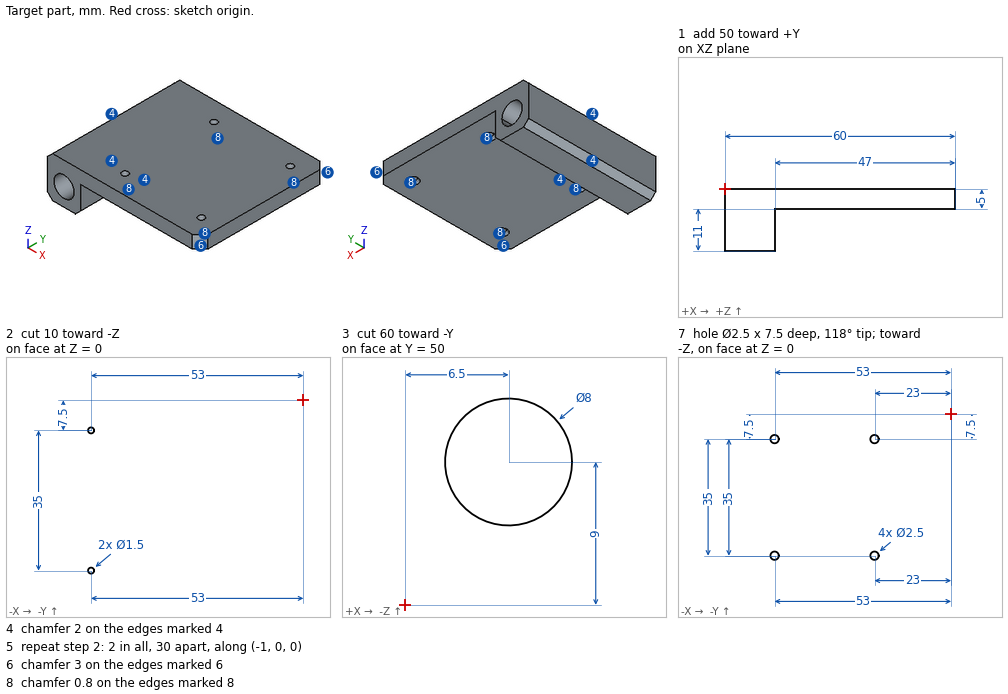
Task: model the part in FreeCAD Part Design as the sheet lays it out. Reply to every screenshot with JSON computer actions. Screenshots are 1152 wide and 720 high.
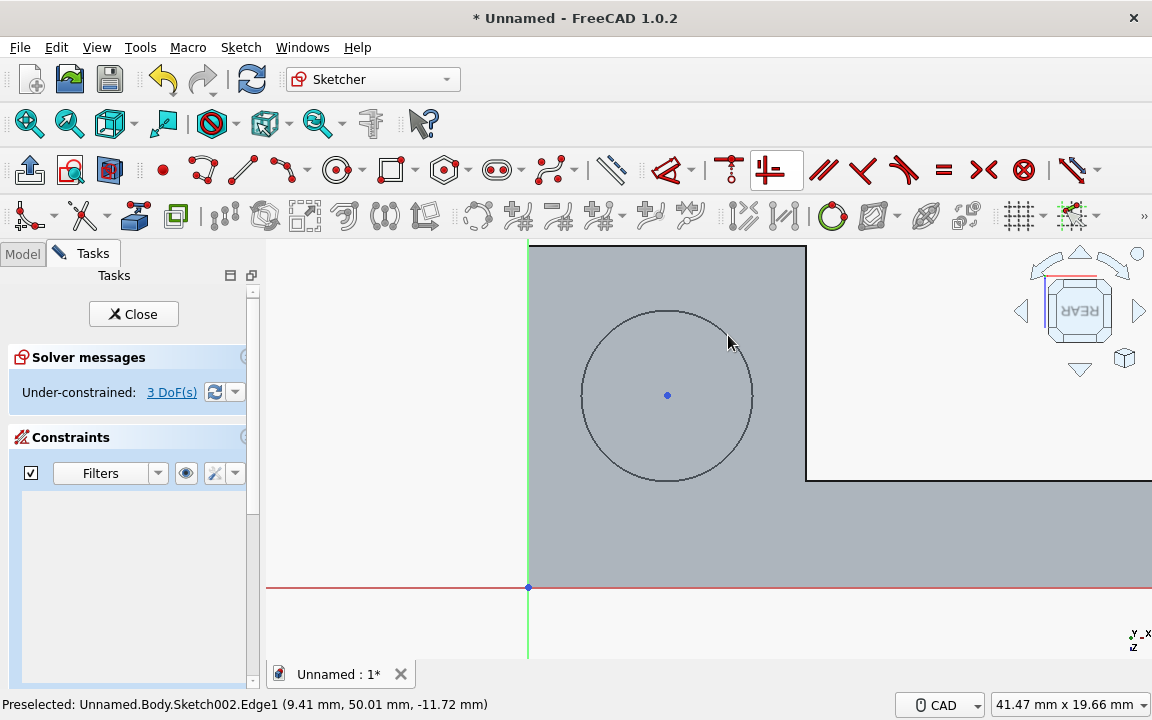
{"action": "left_click", "coordinate": [666, 170]}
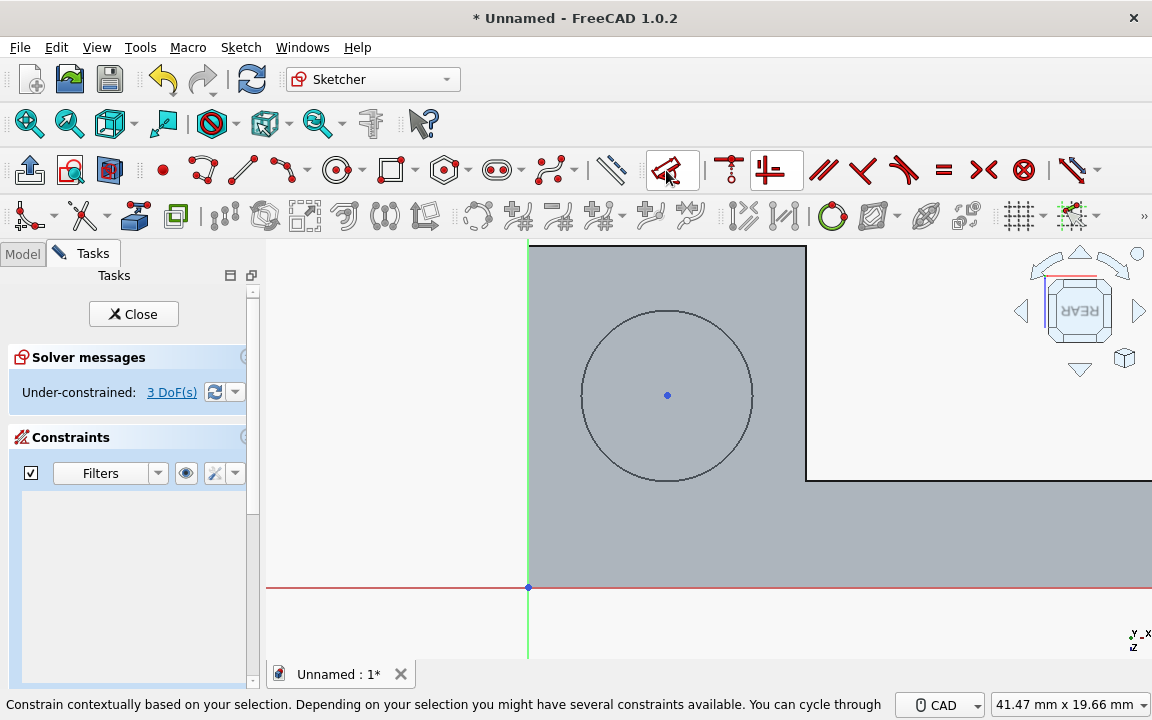
{"action": "left_click", "coordinate": [727, 335]}
{"action": "left_click", "coordinate": [749, 312]}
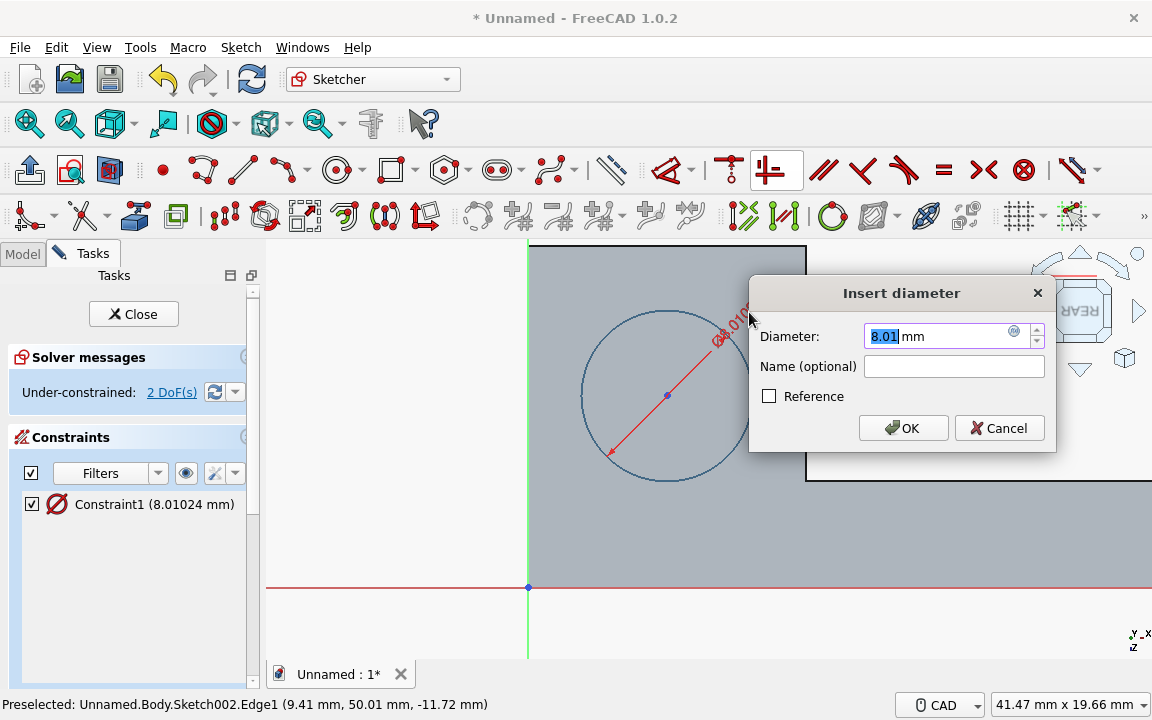
{"action": "type", "text": "8"}
{"action": "key", "text": "Return"}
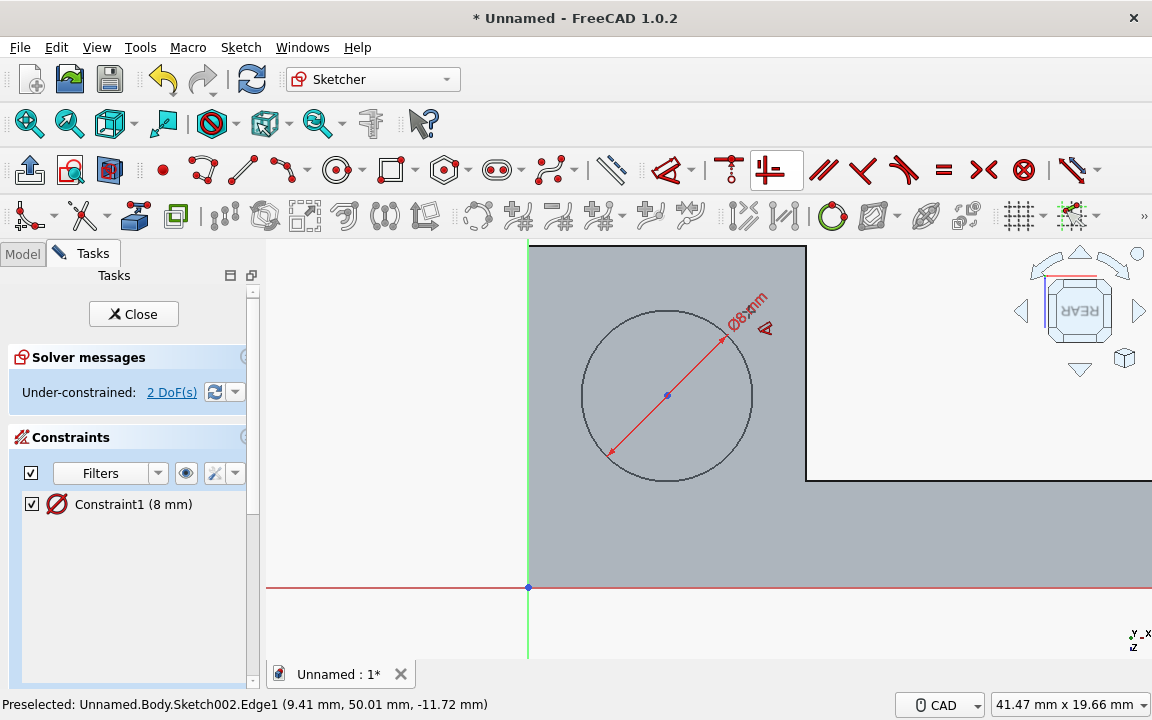
{"action": "left_click", "coordinate": [667, 396]}
{"action": "left_click", "coordinate": [494, 492]}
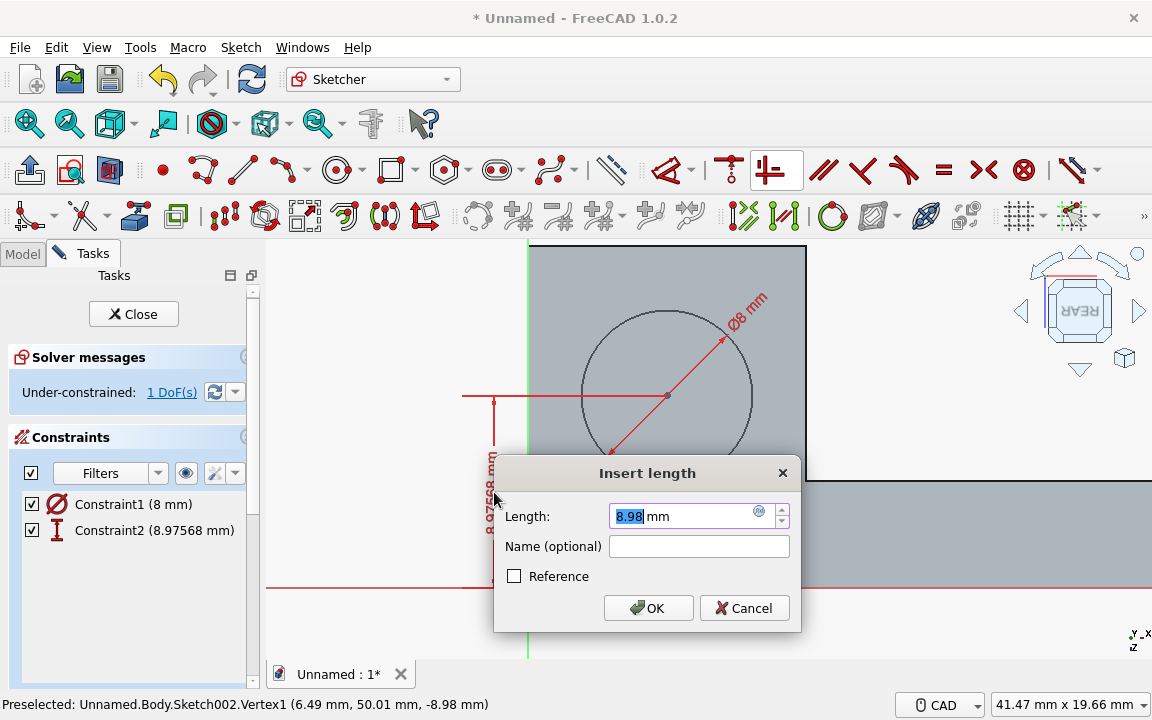
{"action": "type", "text": "9"}
{"action": "key", "text": "Return"}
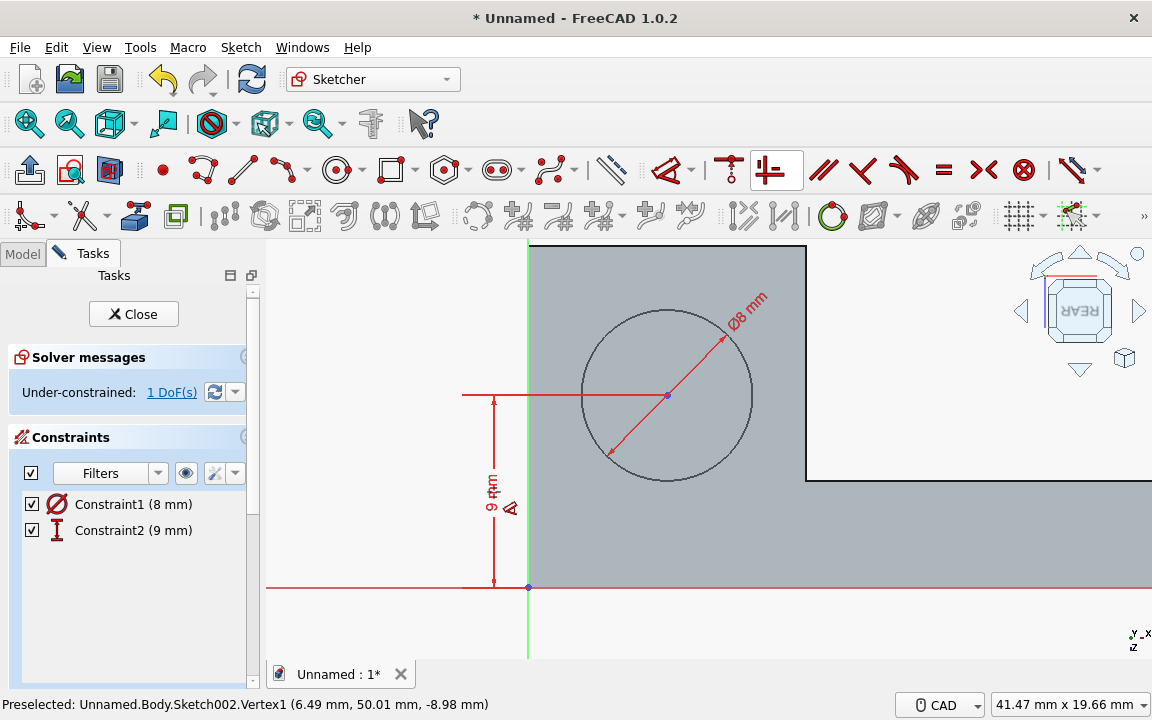
{"action": "left_click", "coordinate": [667, 395]}
{"action": "left_click", "coordinate": [598, 622]}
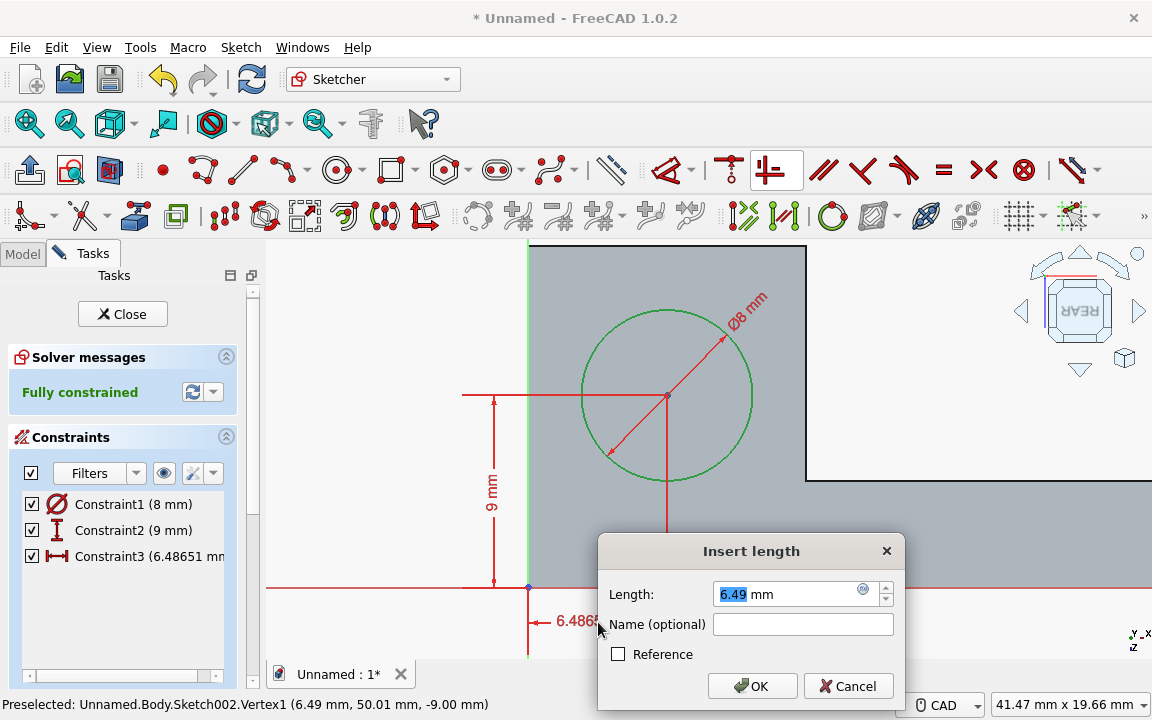
{"action": "type", "text": "6.5"}
{"action": "key", "text": "Return"}
{"action": "key", "text": "Escape"}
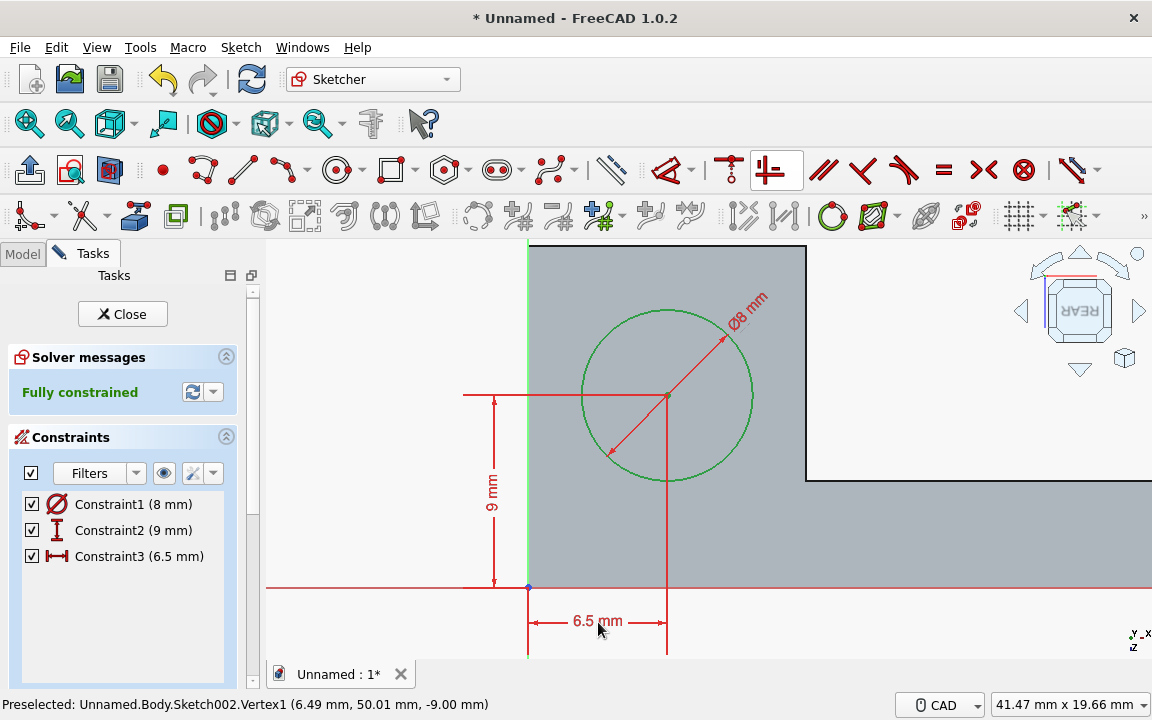
{"action": "left_click", "coordinate": [123, 314]}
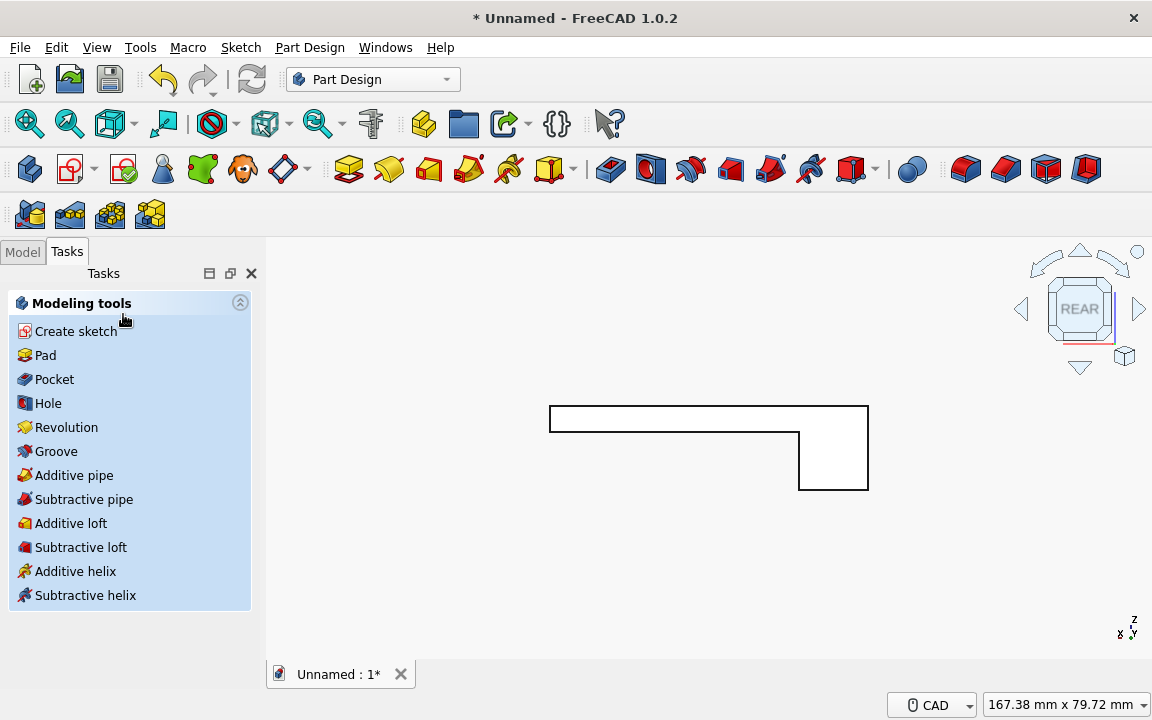
{"action": "left_click", "coordinate": [612, 170]}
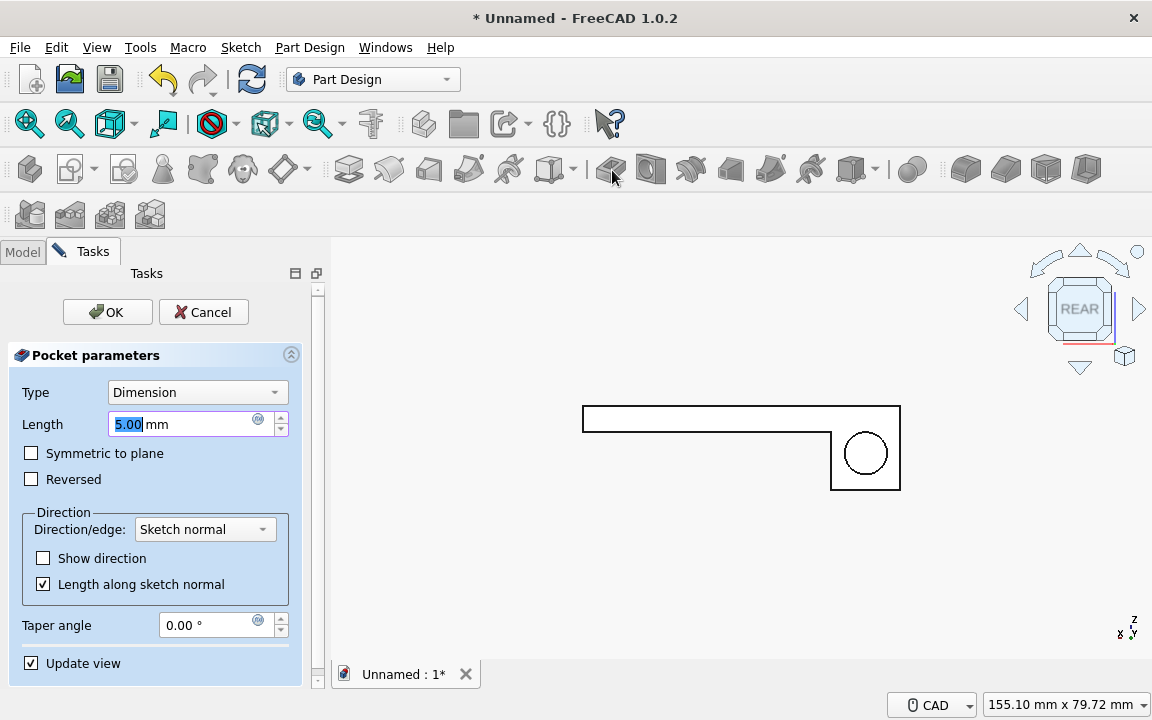
{"action": "type", "text": "60"}
{"action": "key", "text": "Tab"}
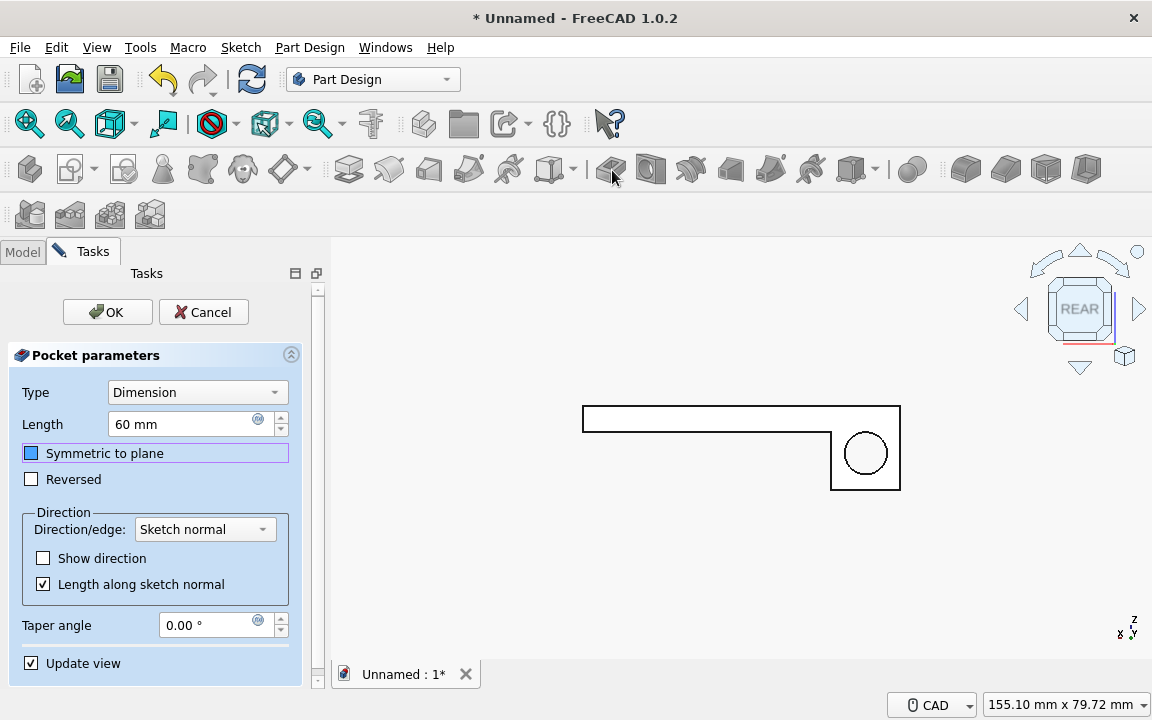
{"action": "left_click", "coordinate": [108, 312]}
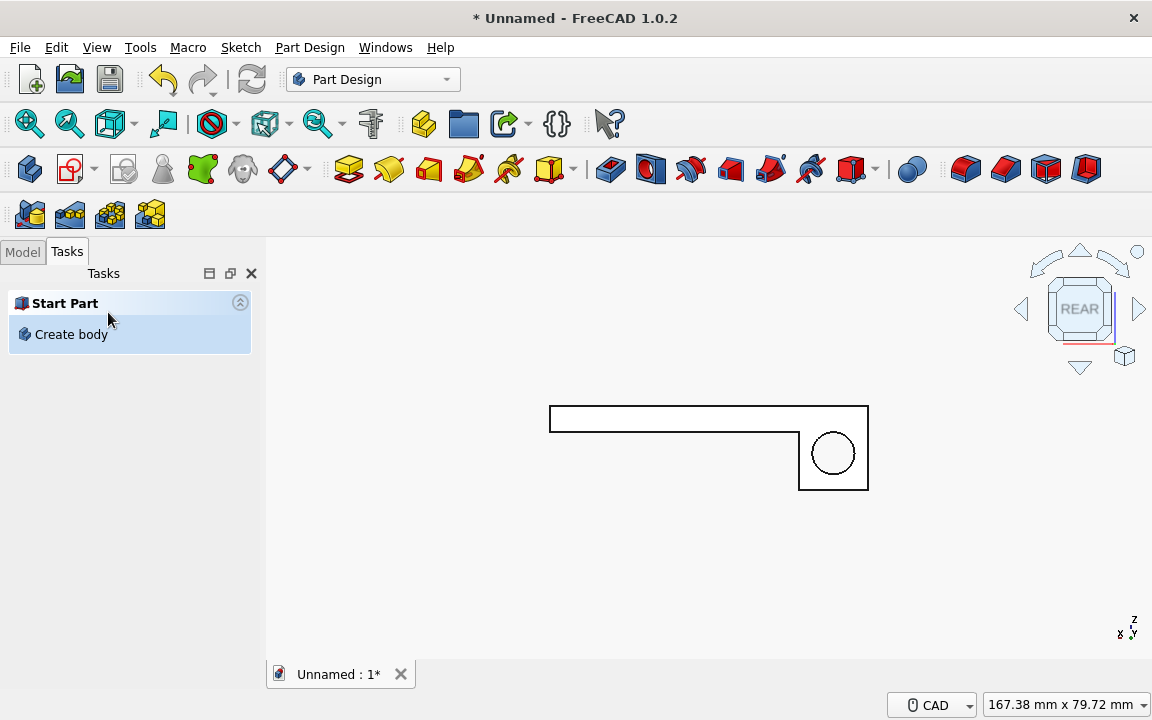
{"action": "key", "text": "v f"}